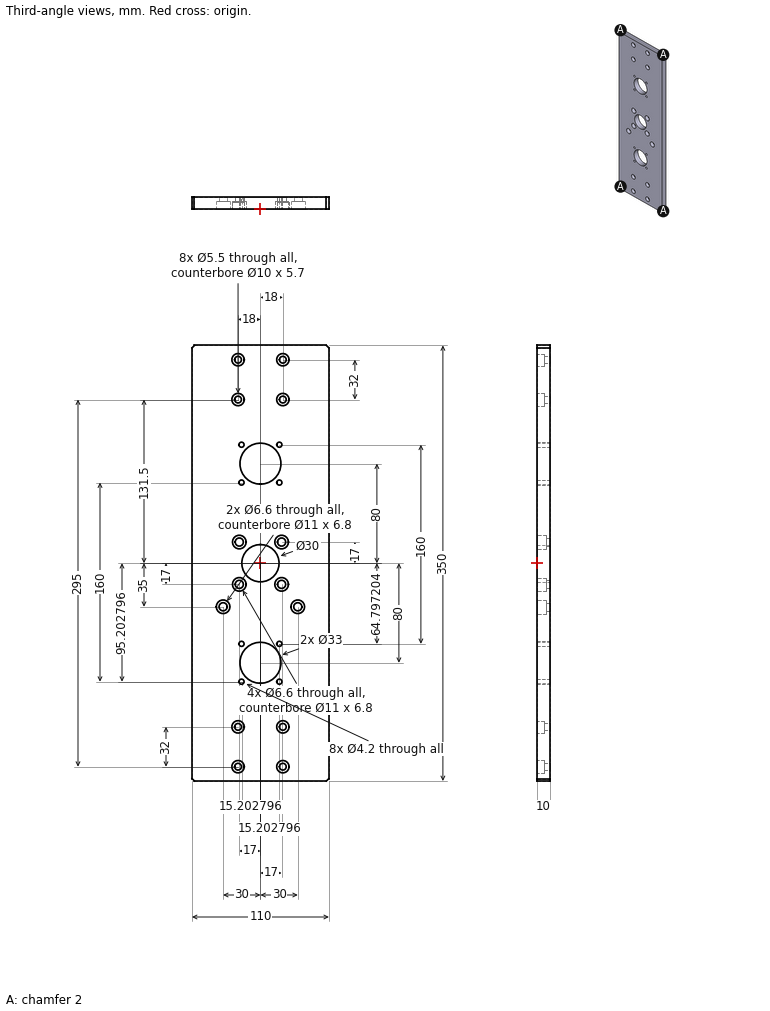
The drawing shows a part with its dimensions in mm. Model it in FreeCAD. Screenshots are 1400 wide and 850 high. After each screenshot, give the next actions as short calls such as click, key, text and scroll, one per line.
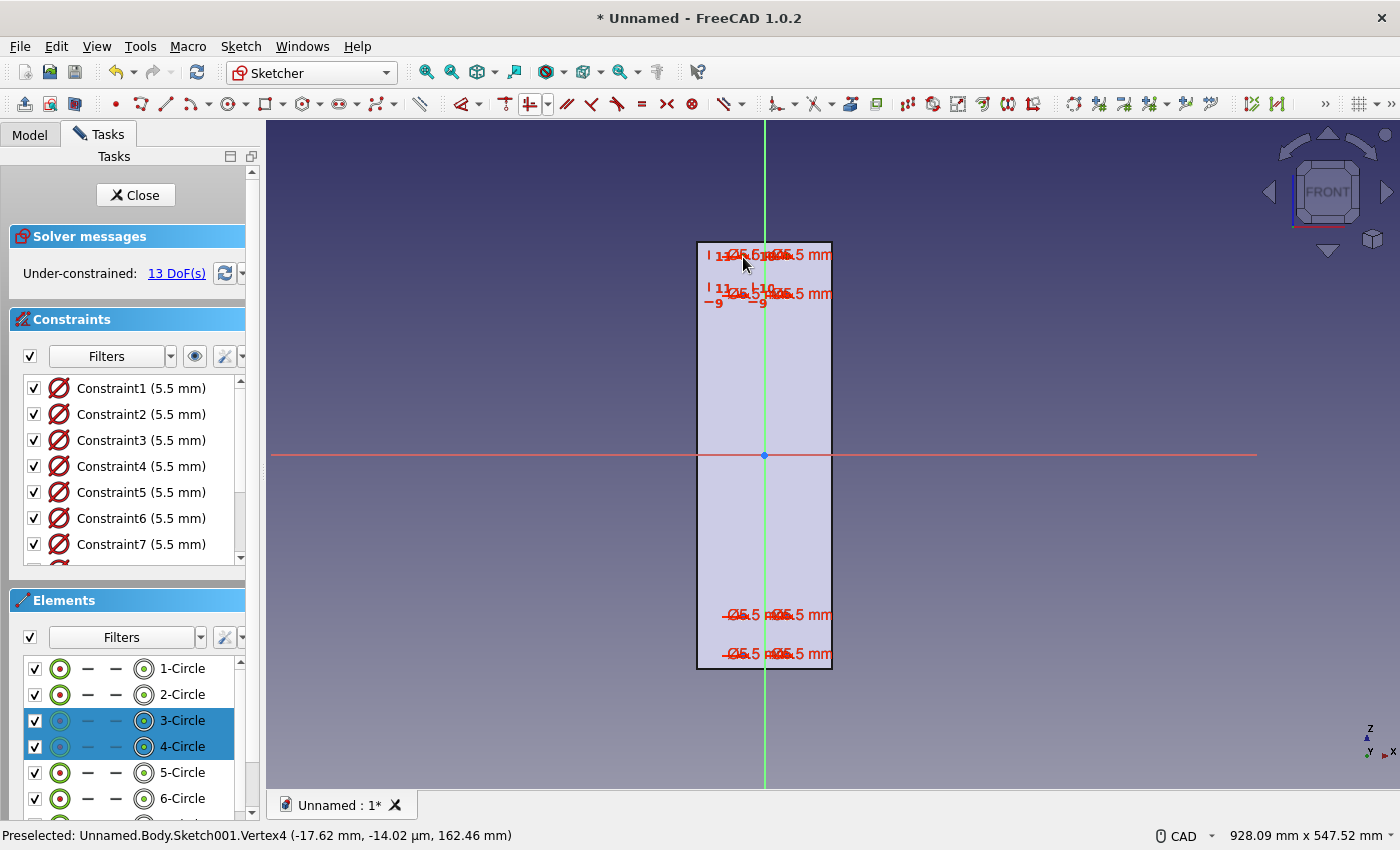
key(h)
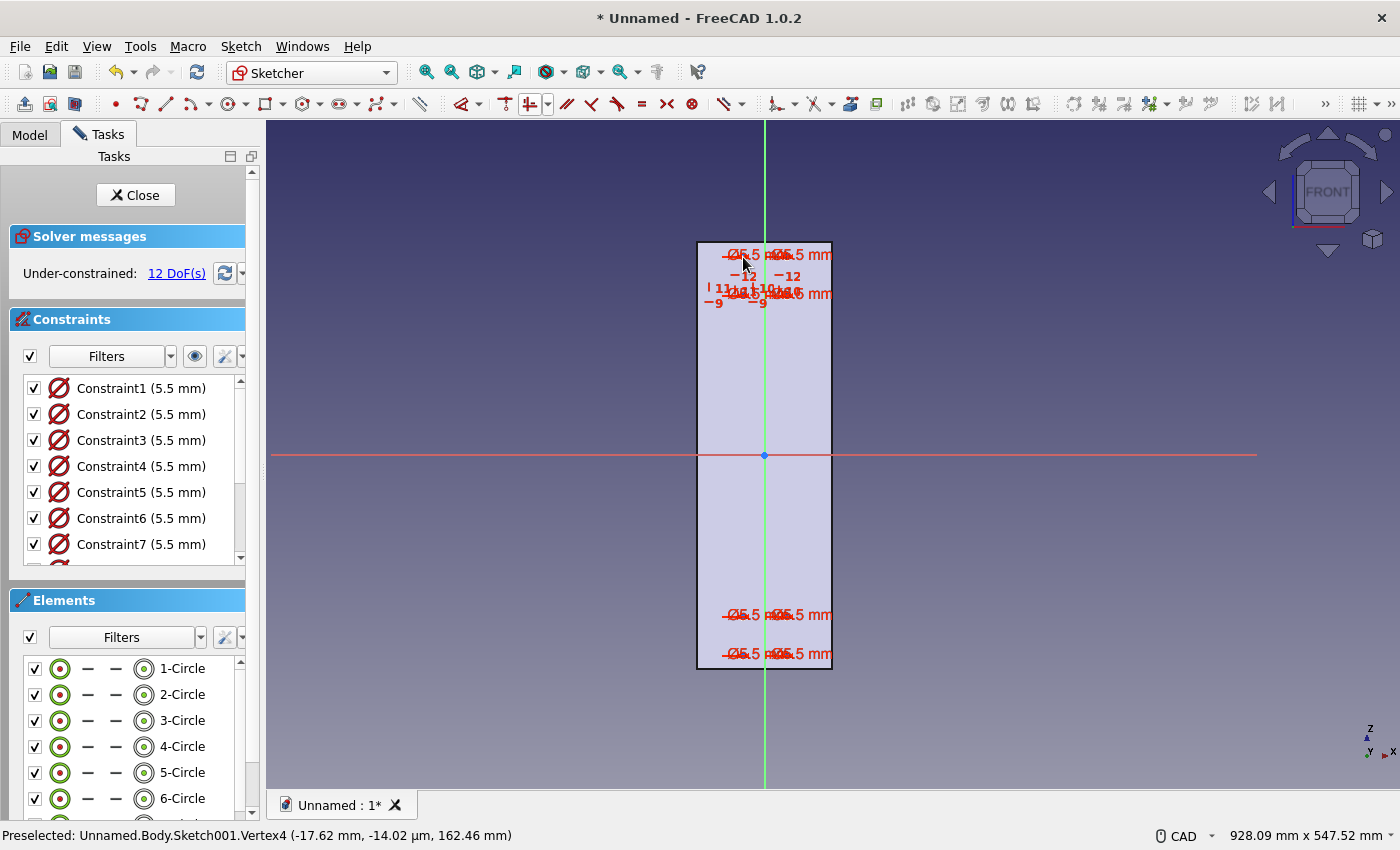
click(741, 298)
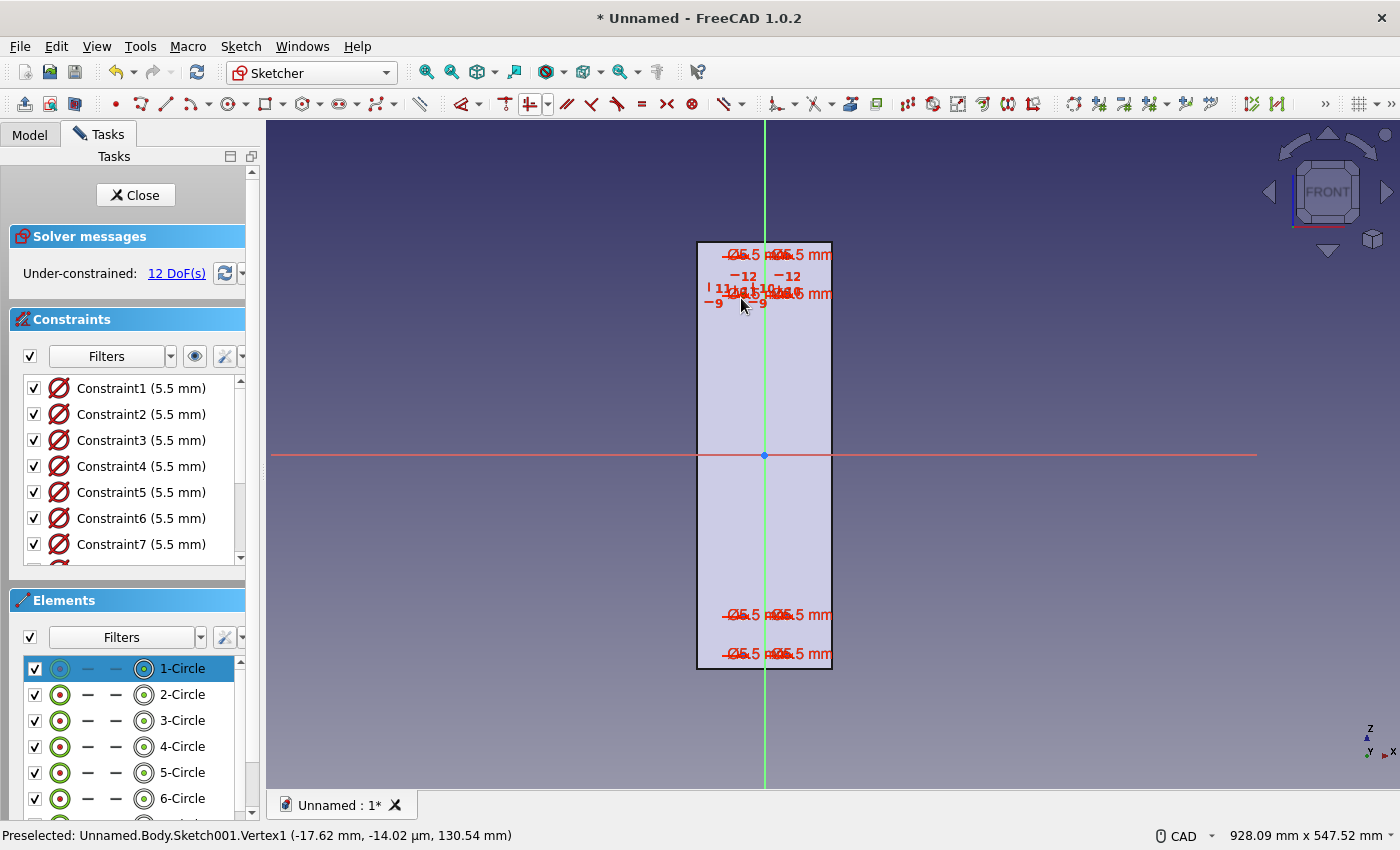
click(743, 656)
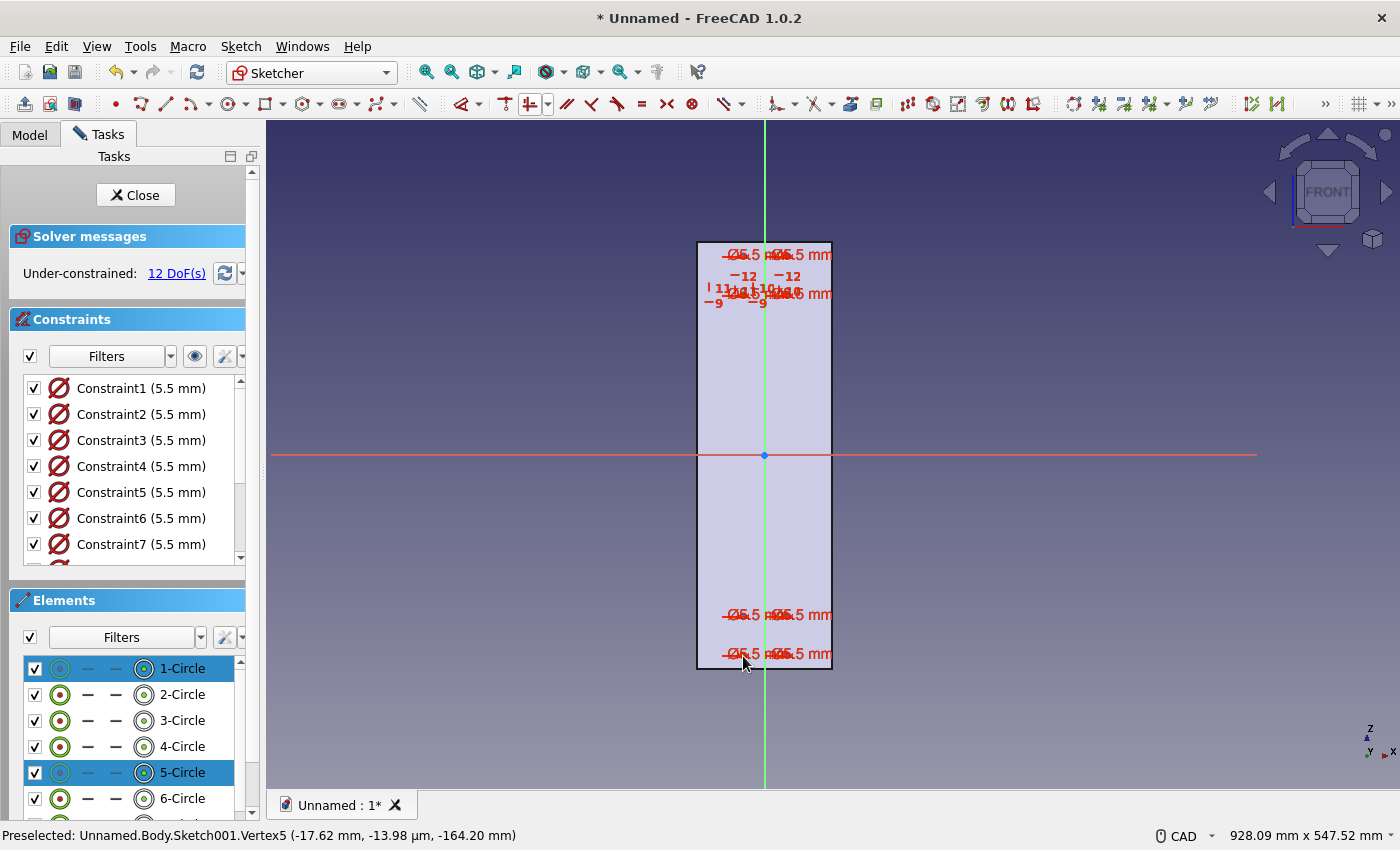
key(v)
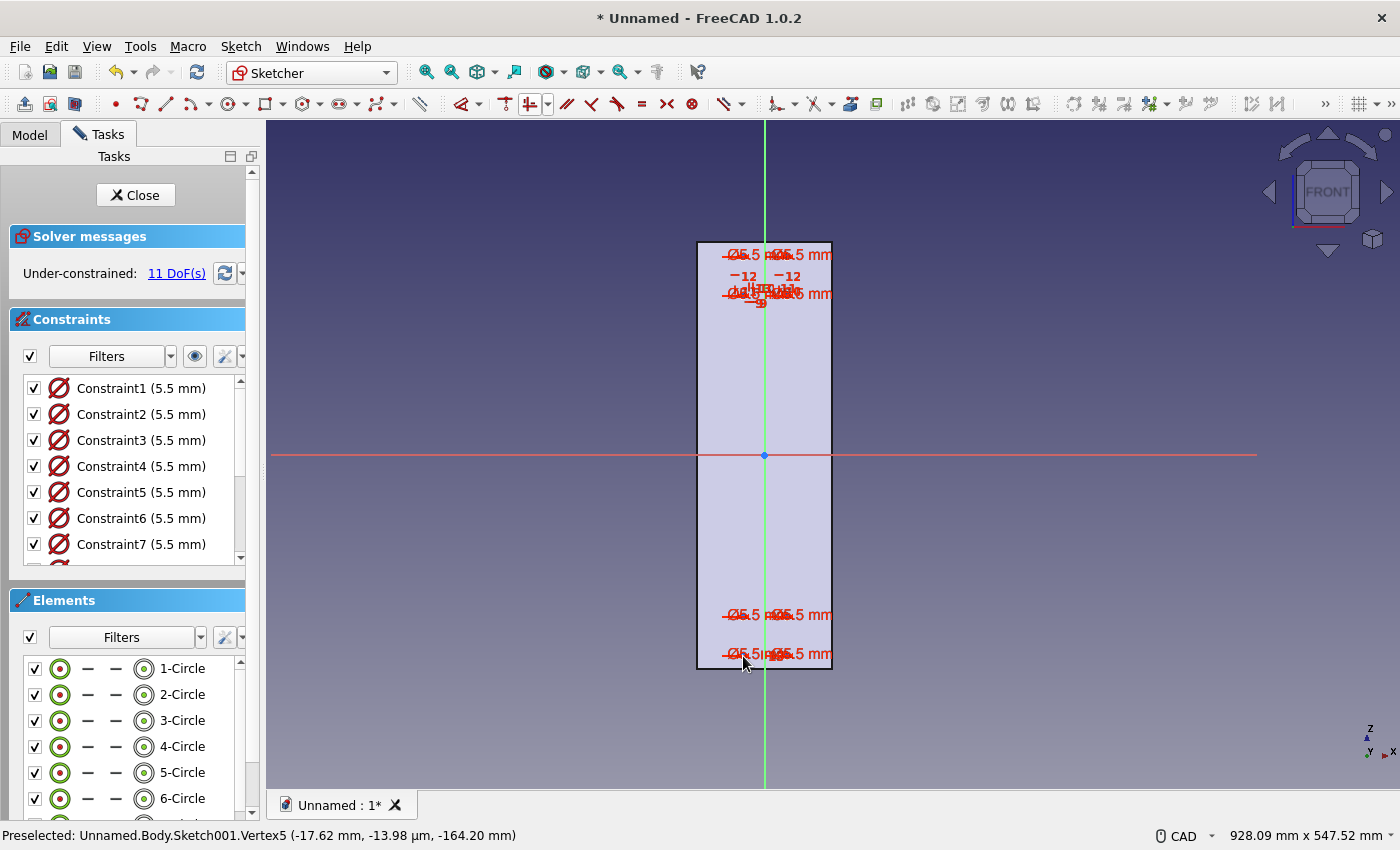
click(743, 656)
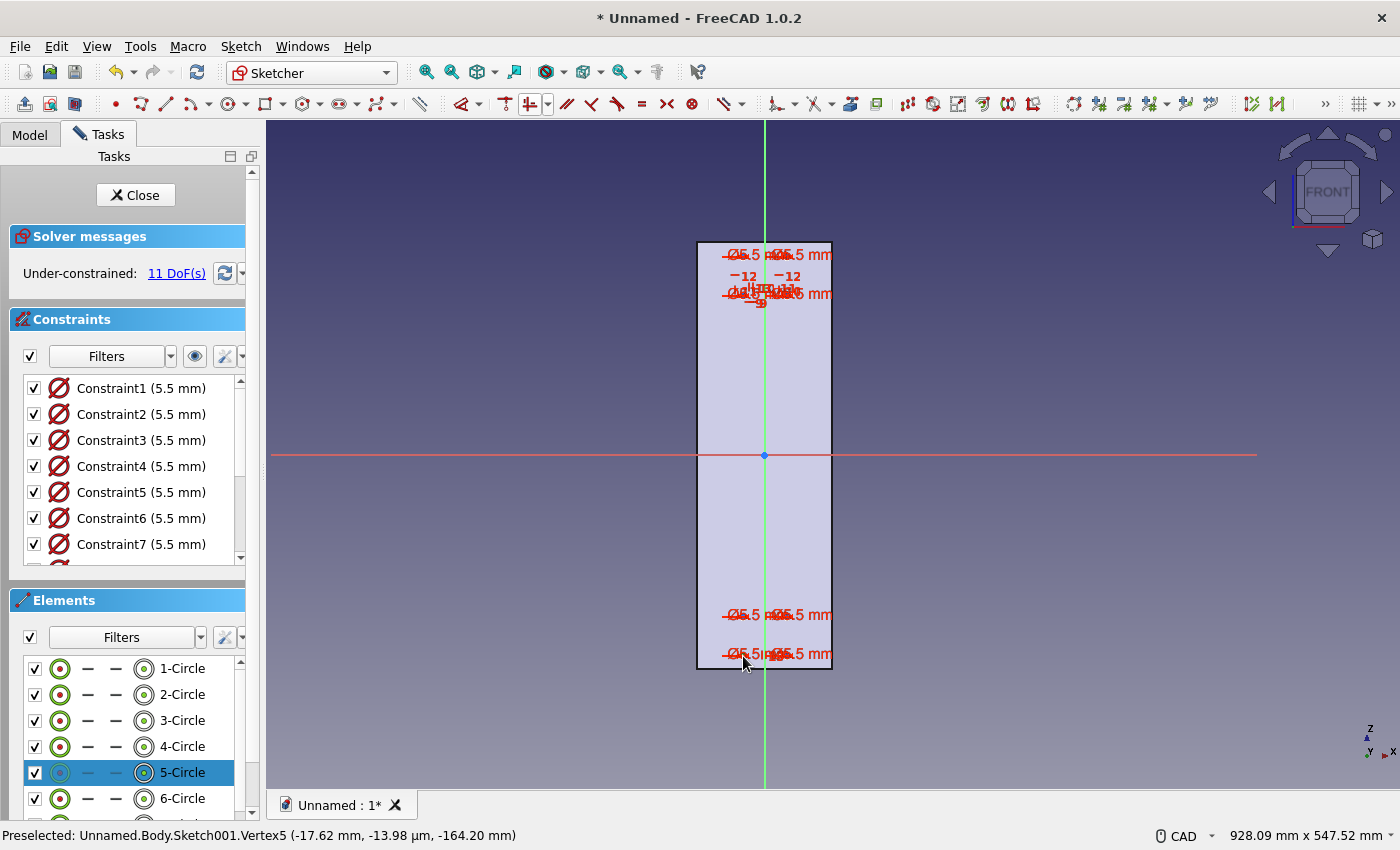
click(743, 617)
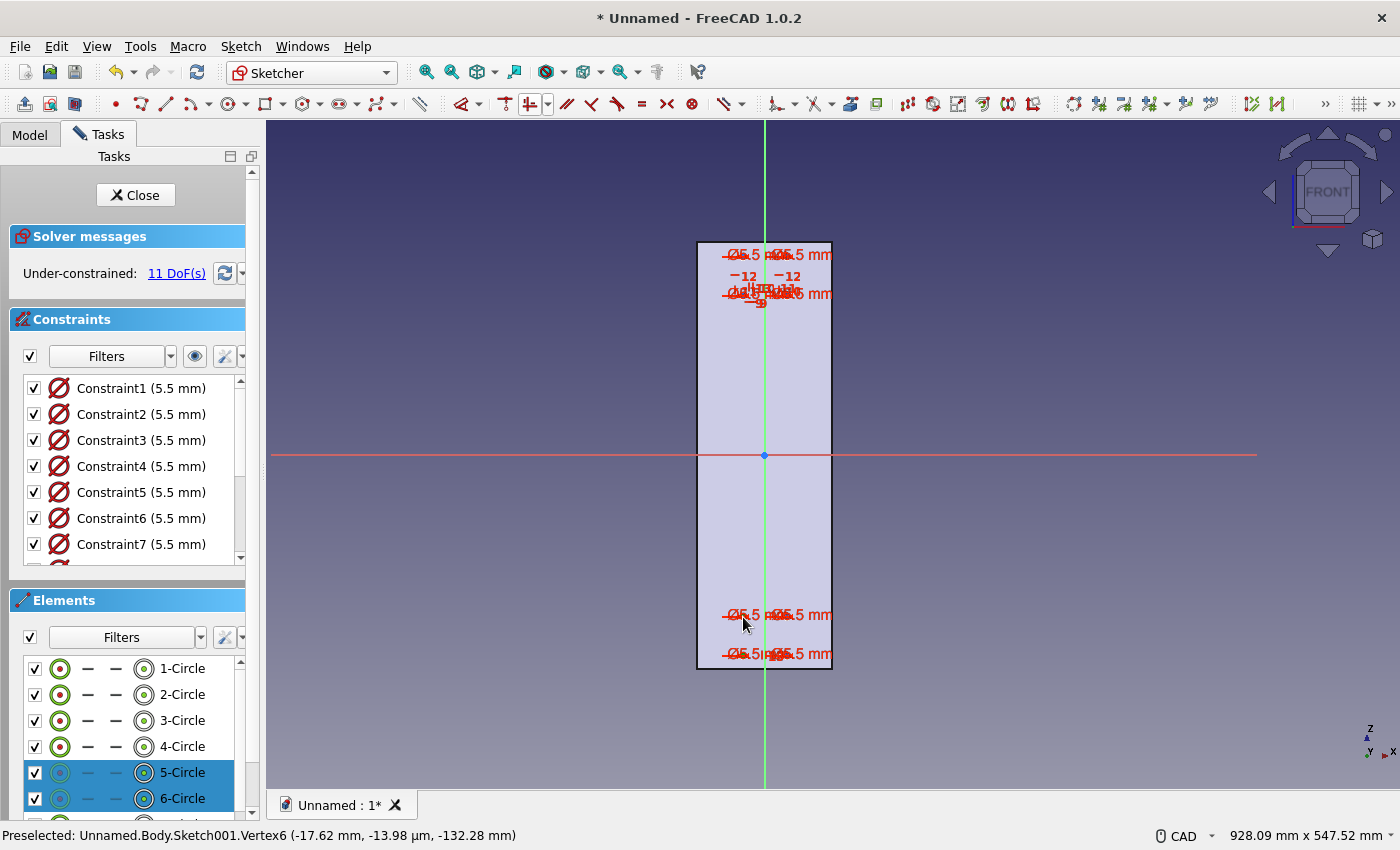
click(548, 104)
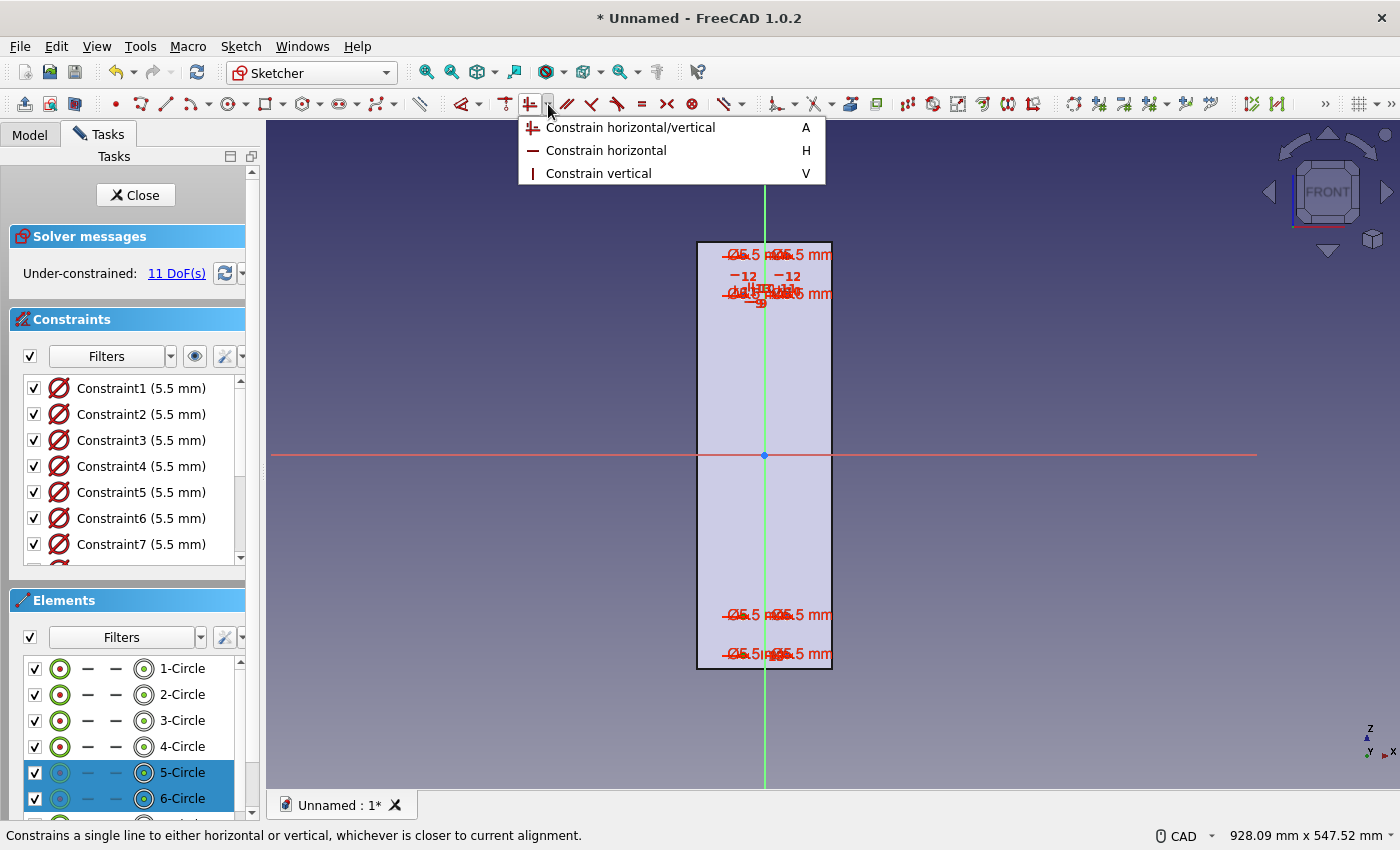
click(672, 174)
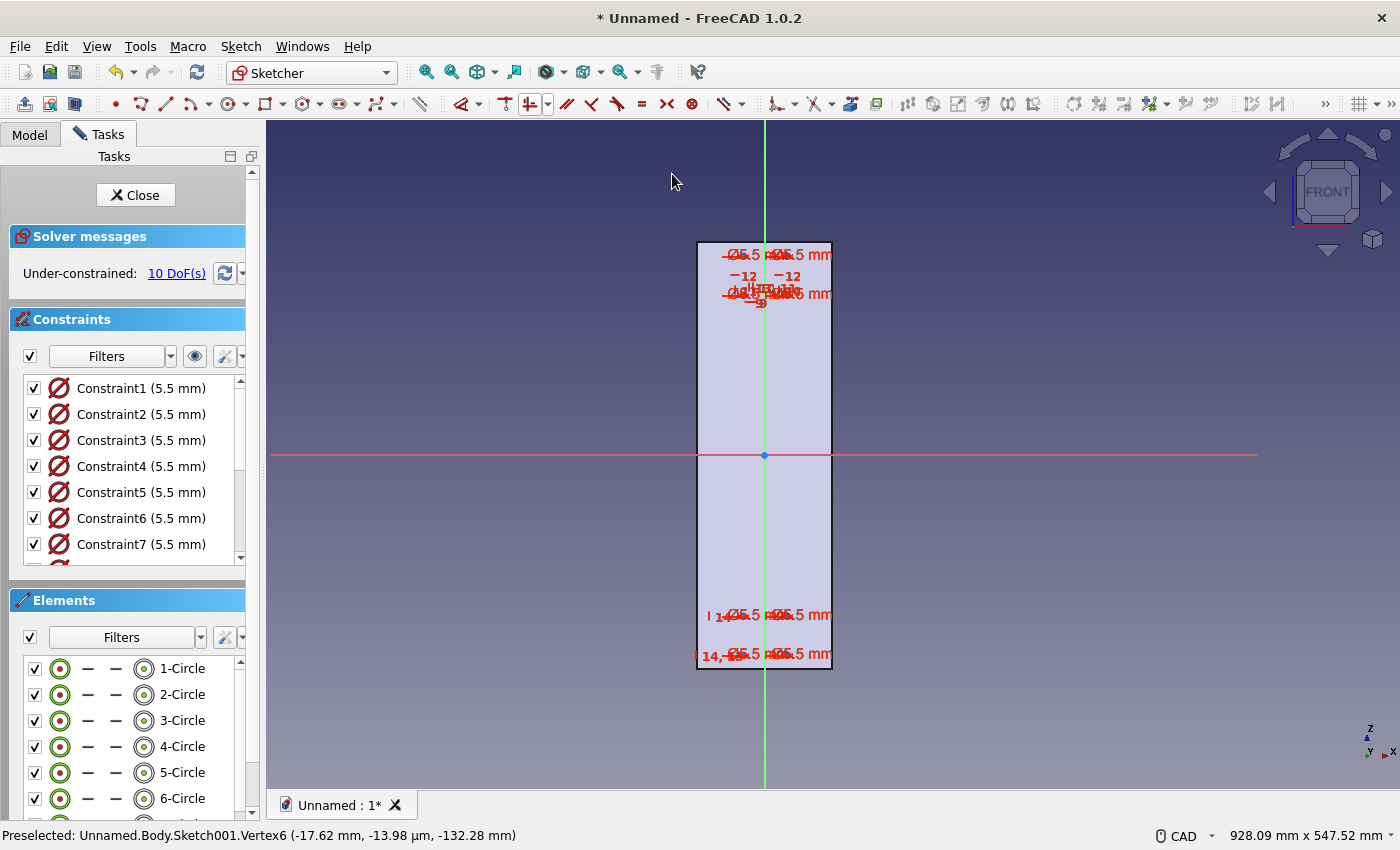
click(787, 296)